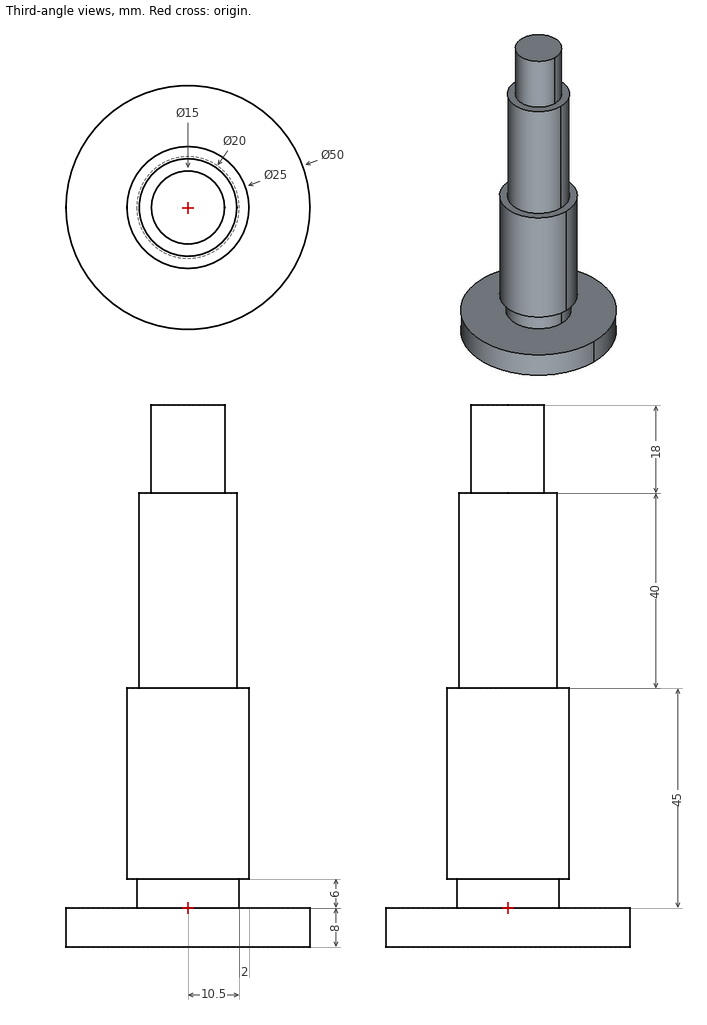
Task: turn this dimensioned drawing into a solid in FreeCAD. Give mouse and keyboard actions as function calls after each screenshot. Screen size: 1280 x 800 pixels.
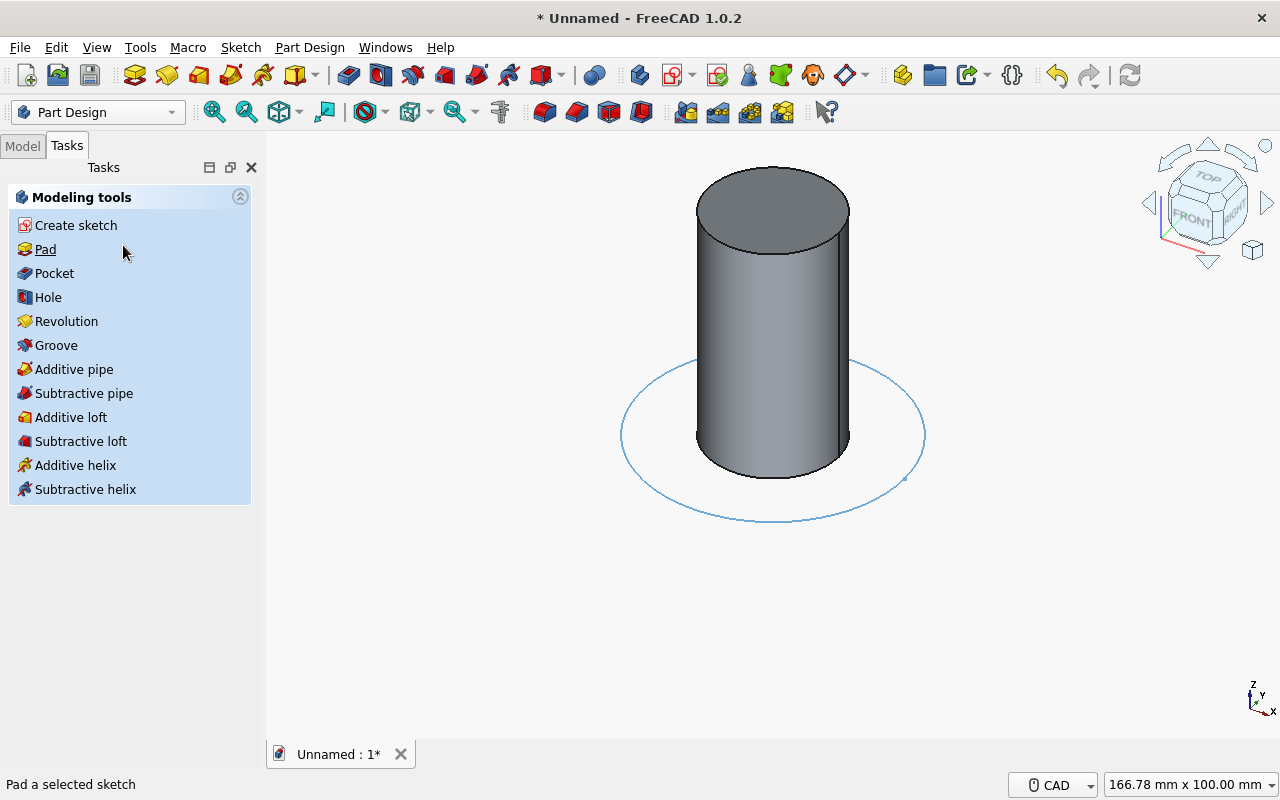
click(136, 76)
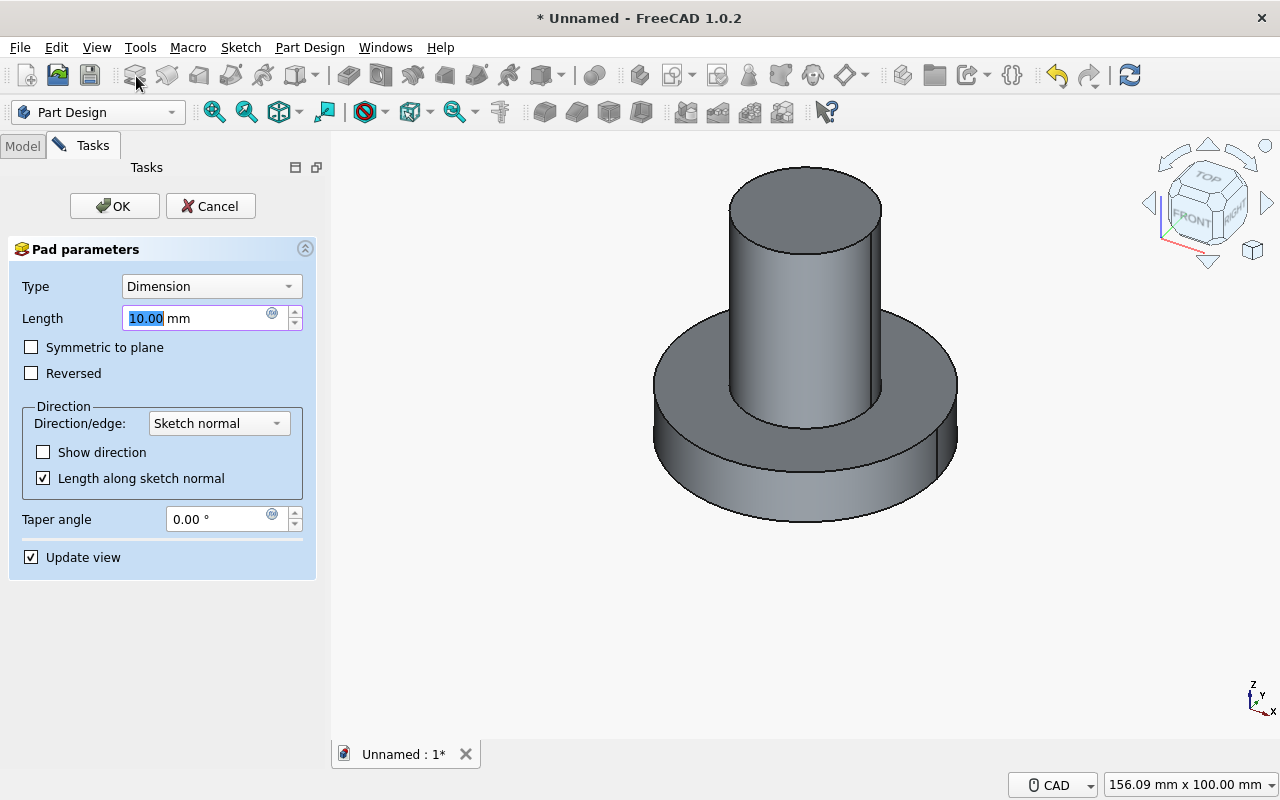
text(8)
key(Tab)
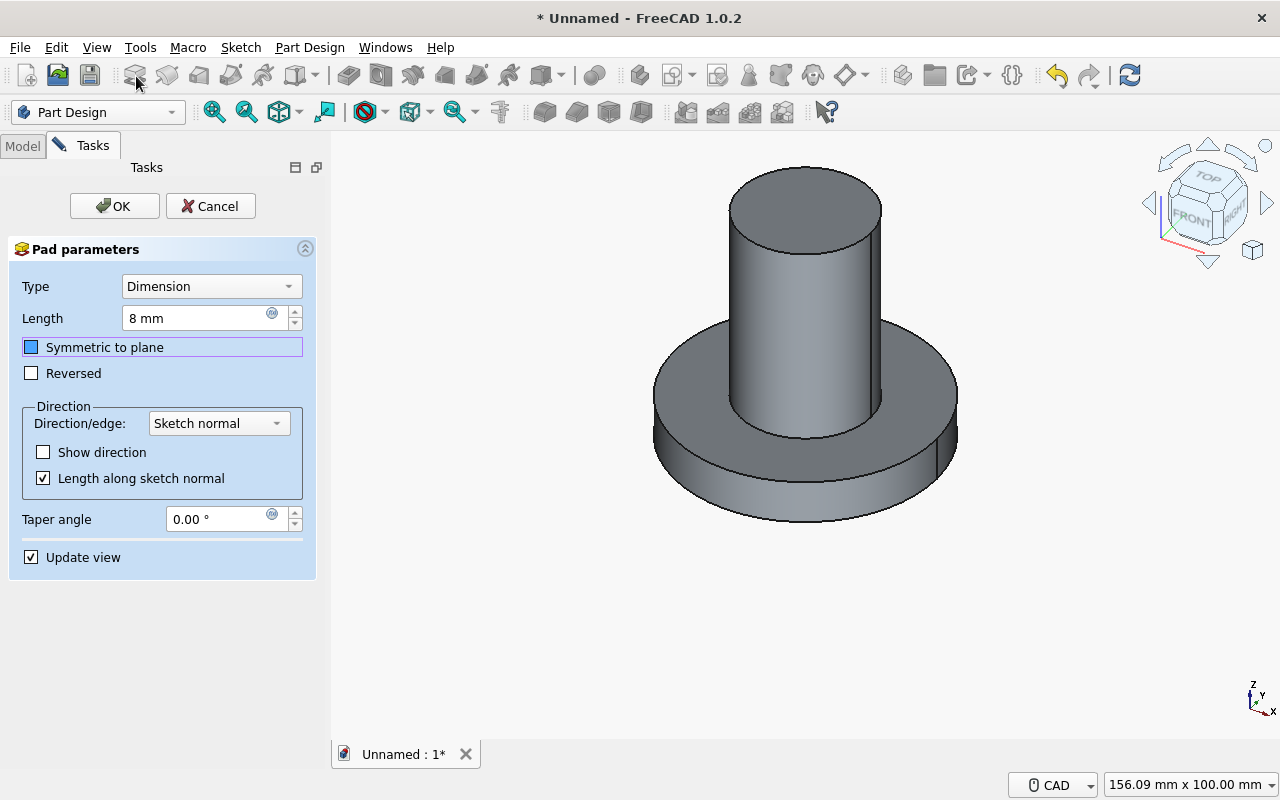
click(30, 373)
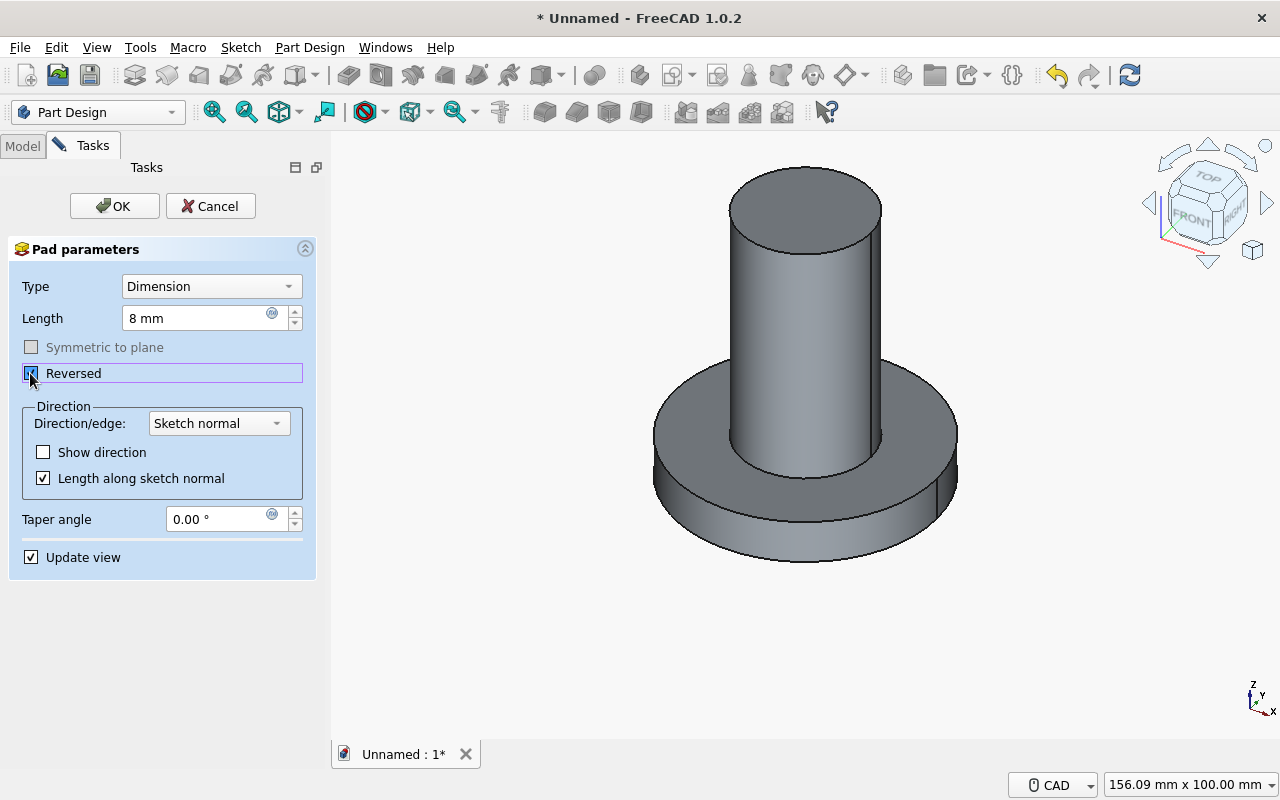
click(115, 206)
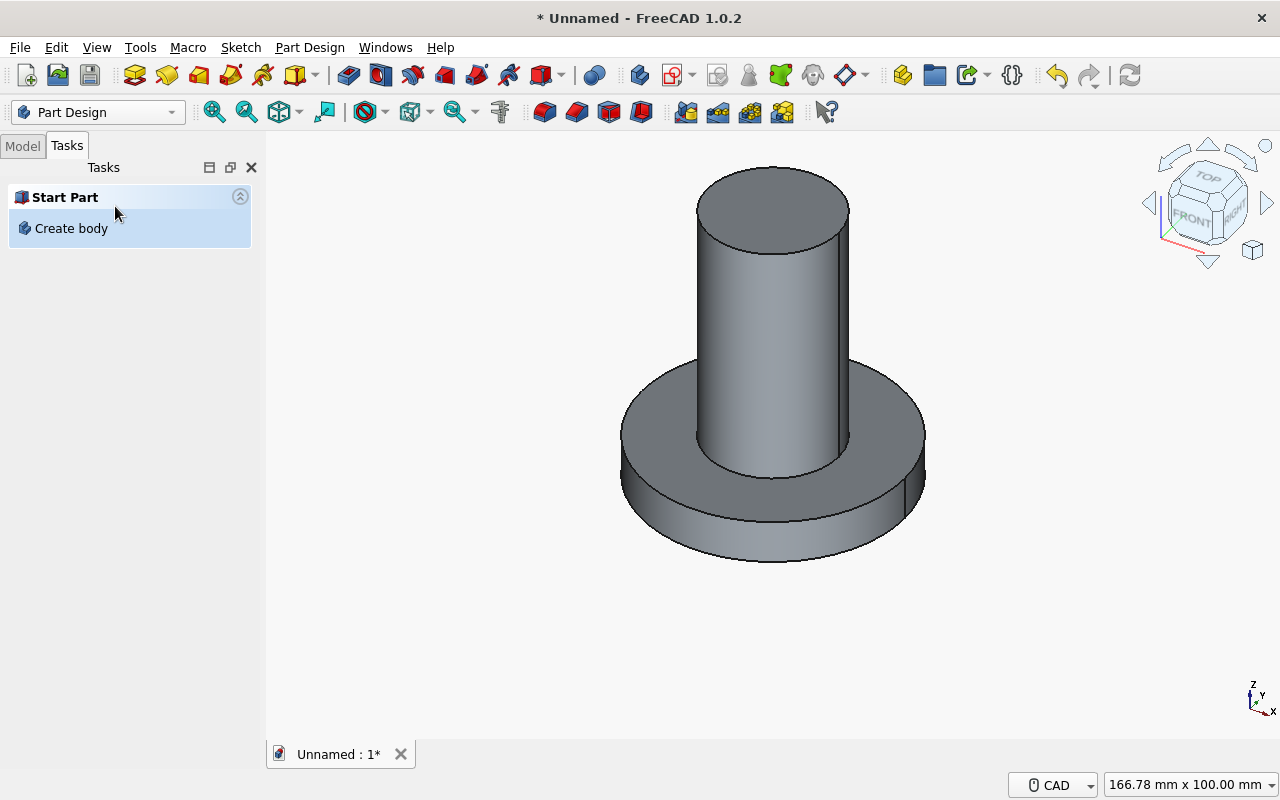
key(v)
key(f)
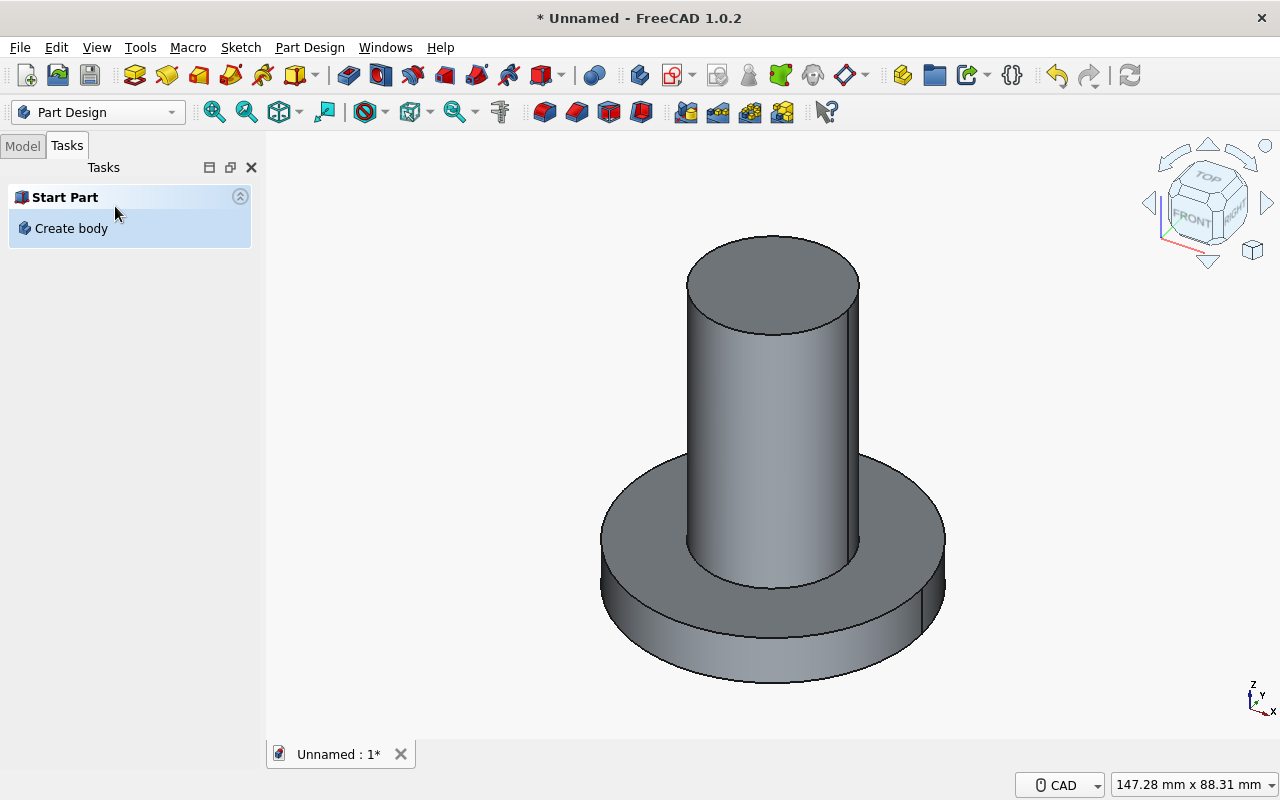
click(773, 285)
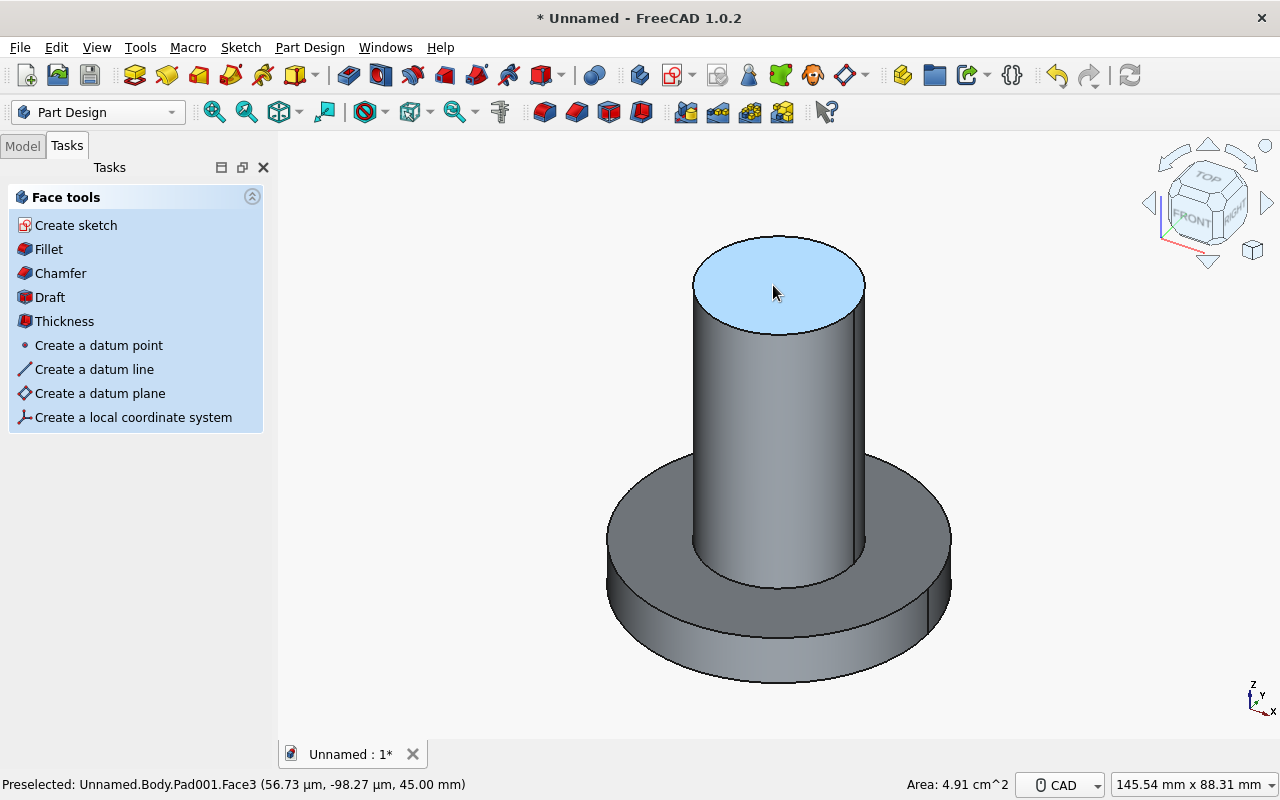
click(672, 76)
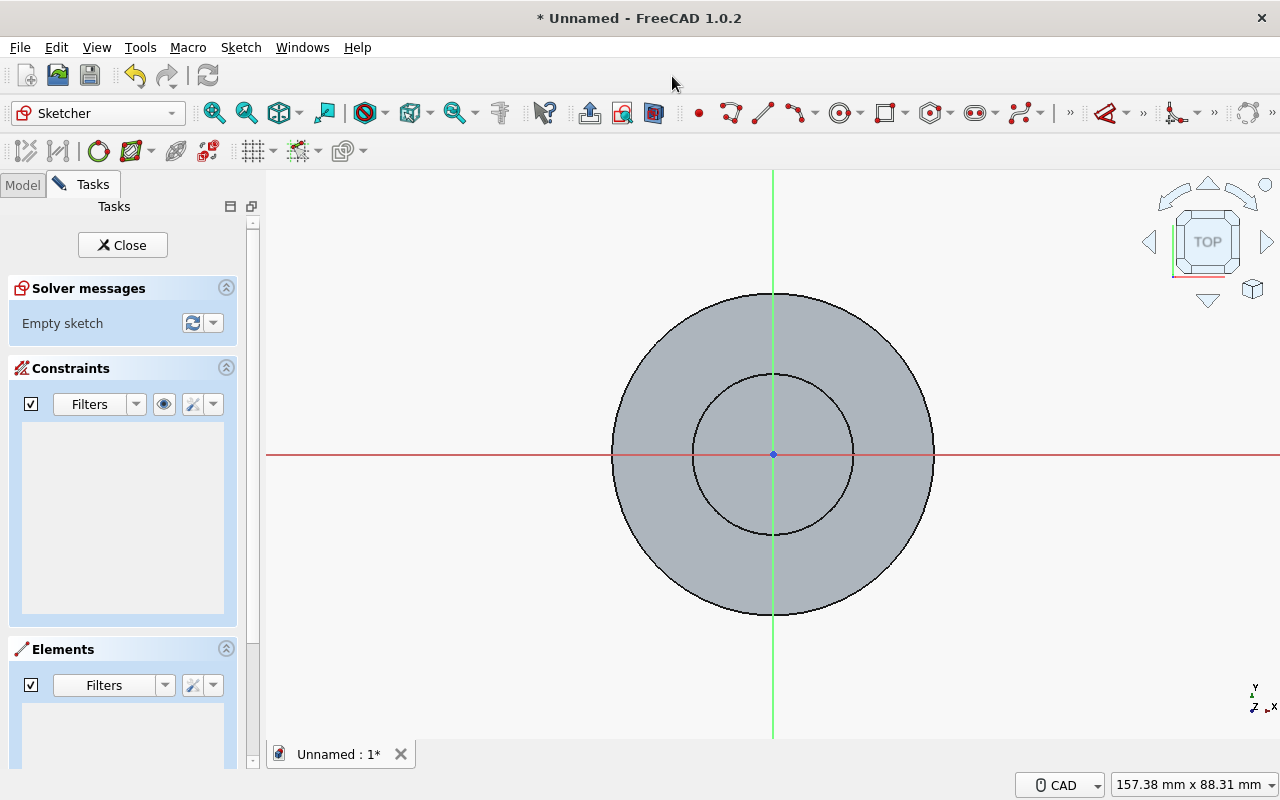
scroll(813, 454, up, 5)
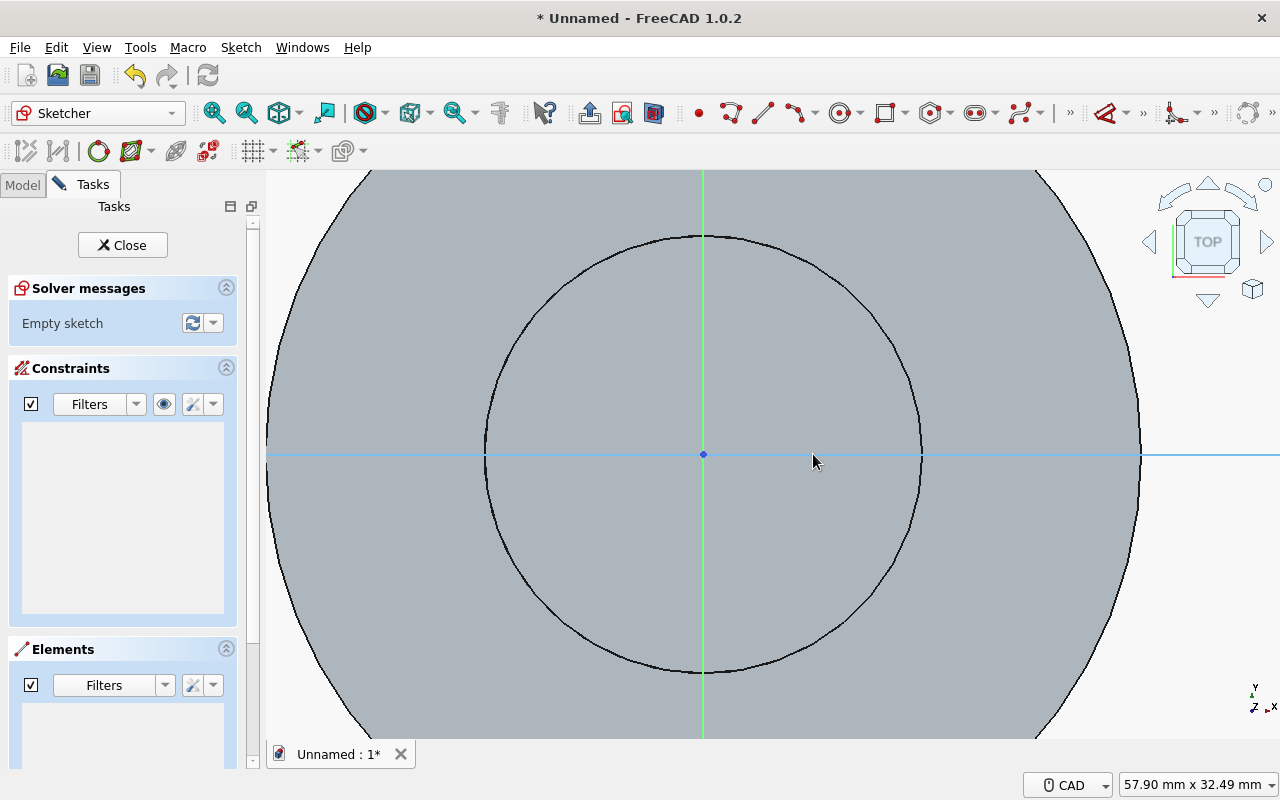
click(840, 114)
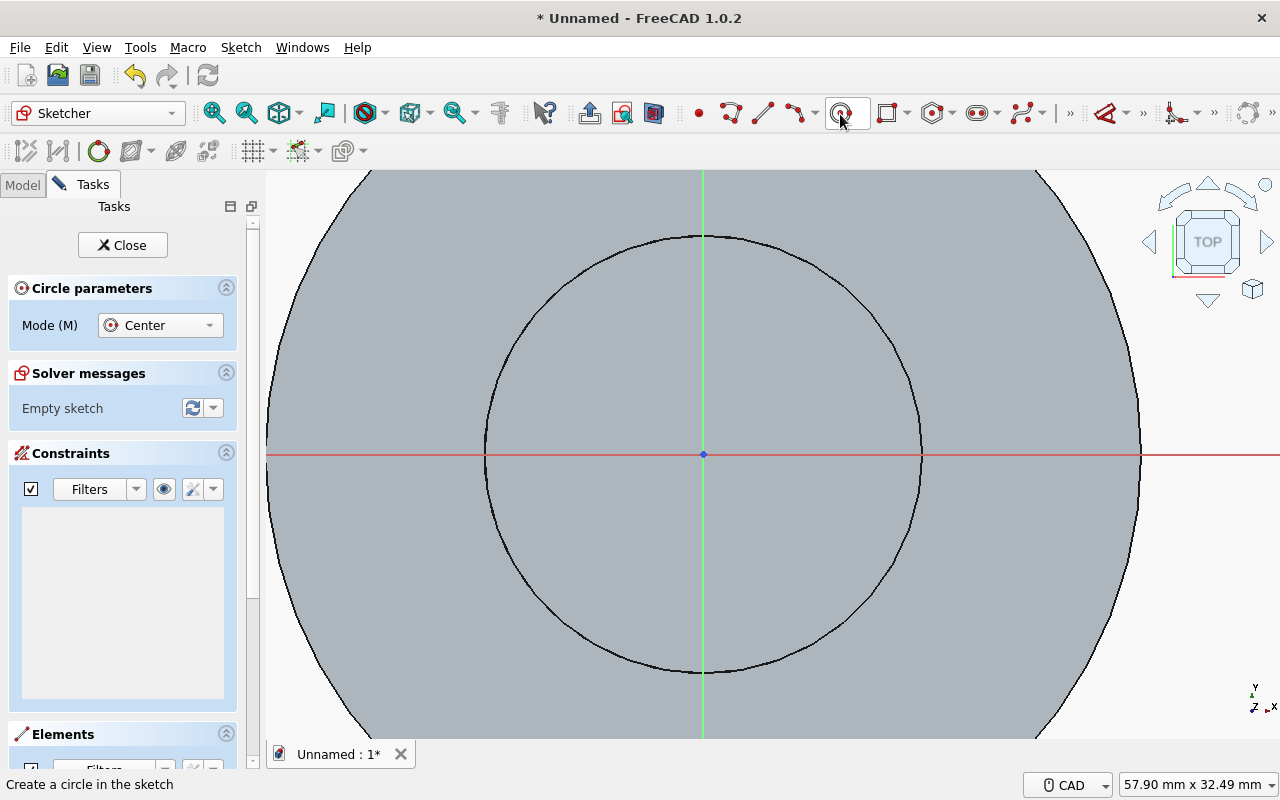
click(703, 454)
move(827, 331)